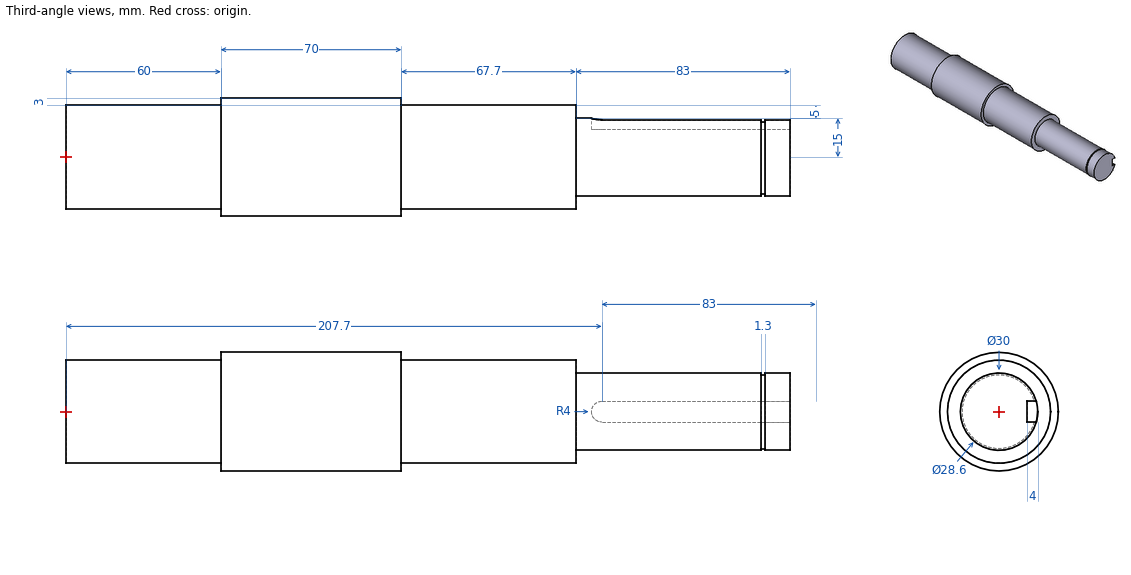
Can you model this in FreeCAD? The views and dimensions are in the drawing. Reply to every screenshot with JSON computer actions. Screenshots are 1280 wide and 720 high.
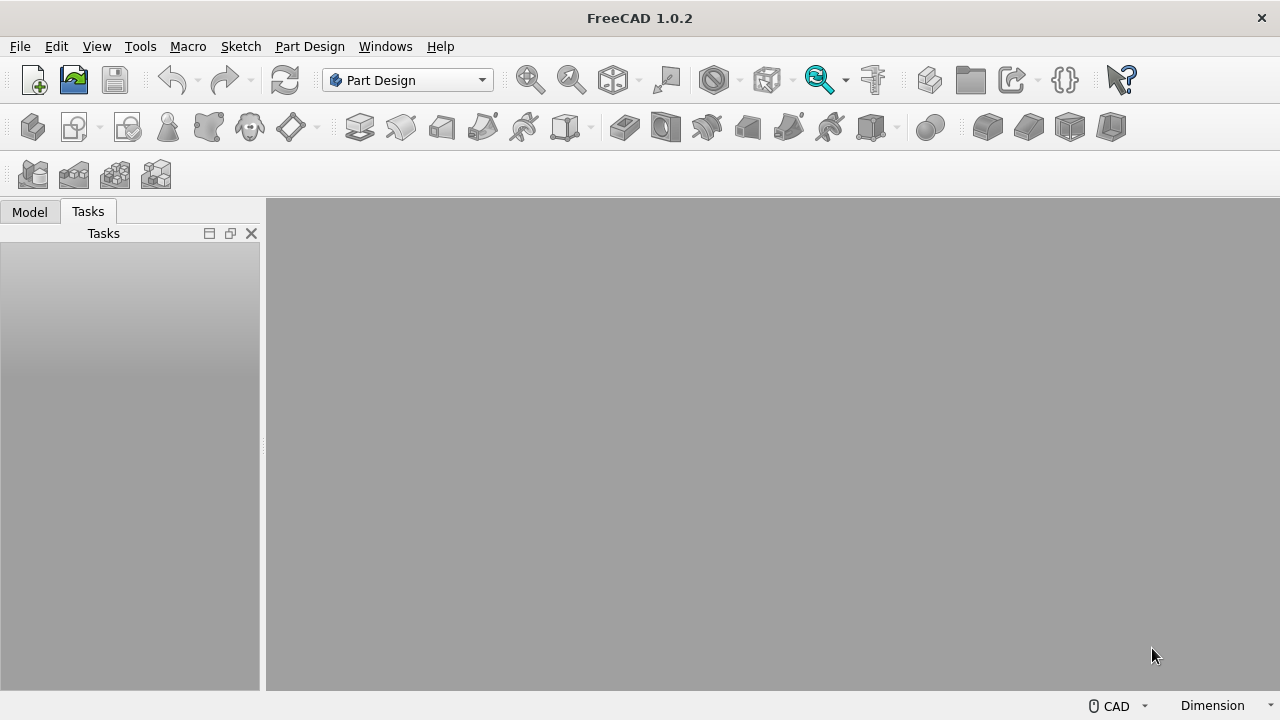
{"action": "key", "text": "ctrl+n"}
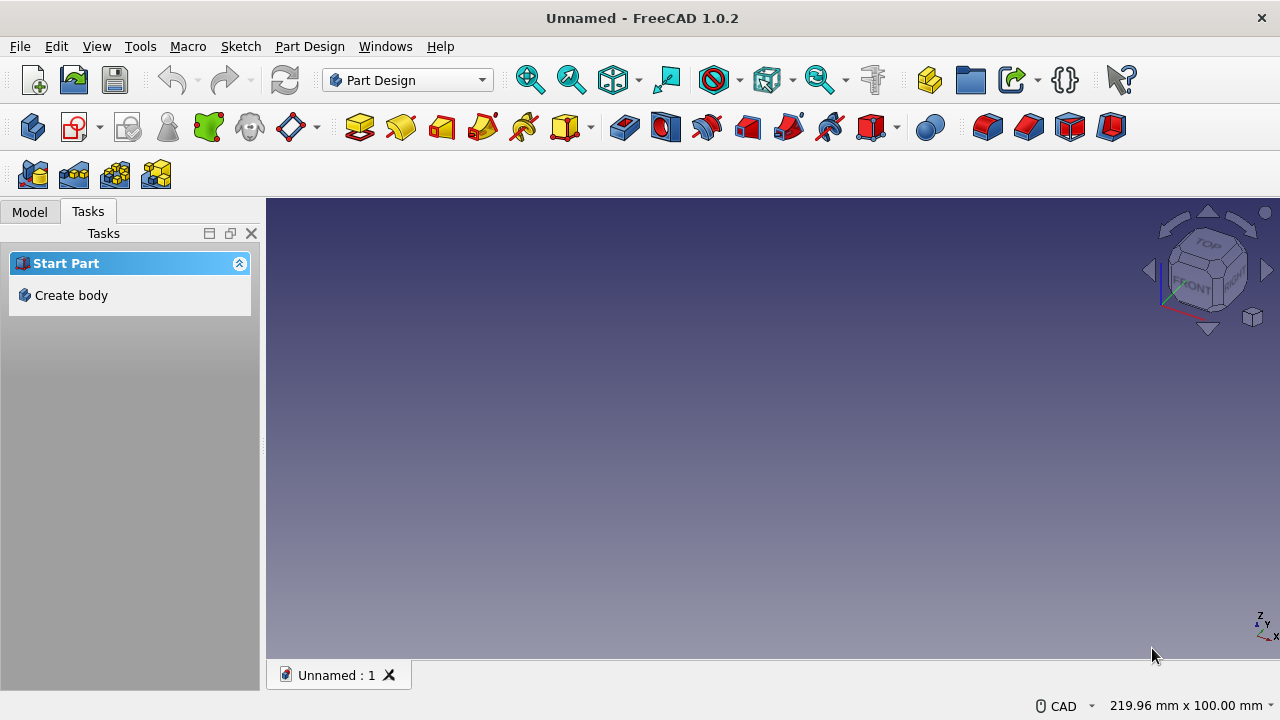
{"action": "left_click", "coordinate": [74, 128]}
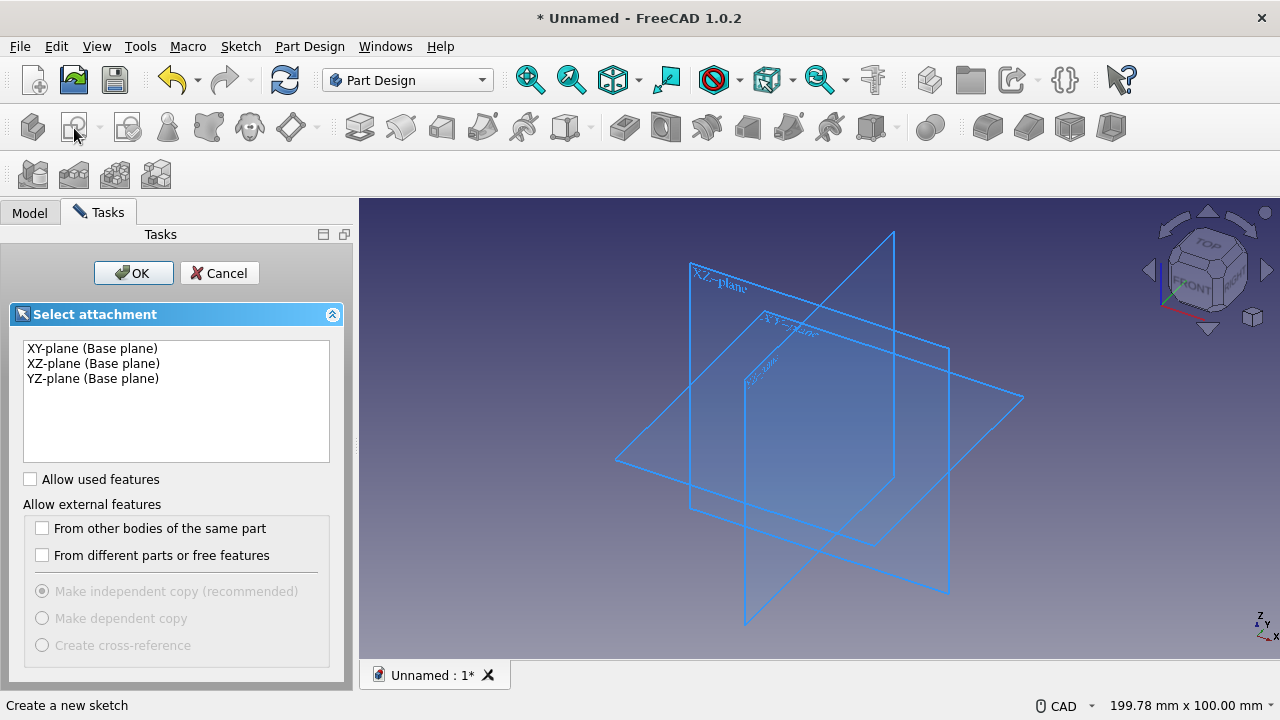
{"action": "left_click", "coordinate": [84, 348]}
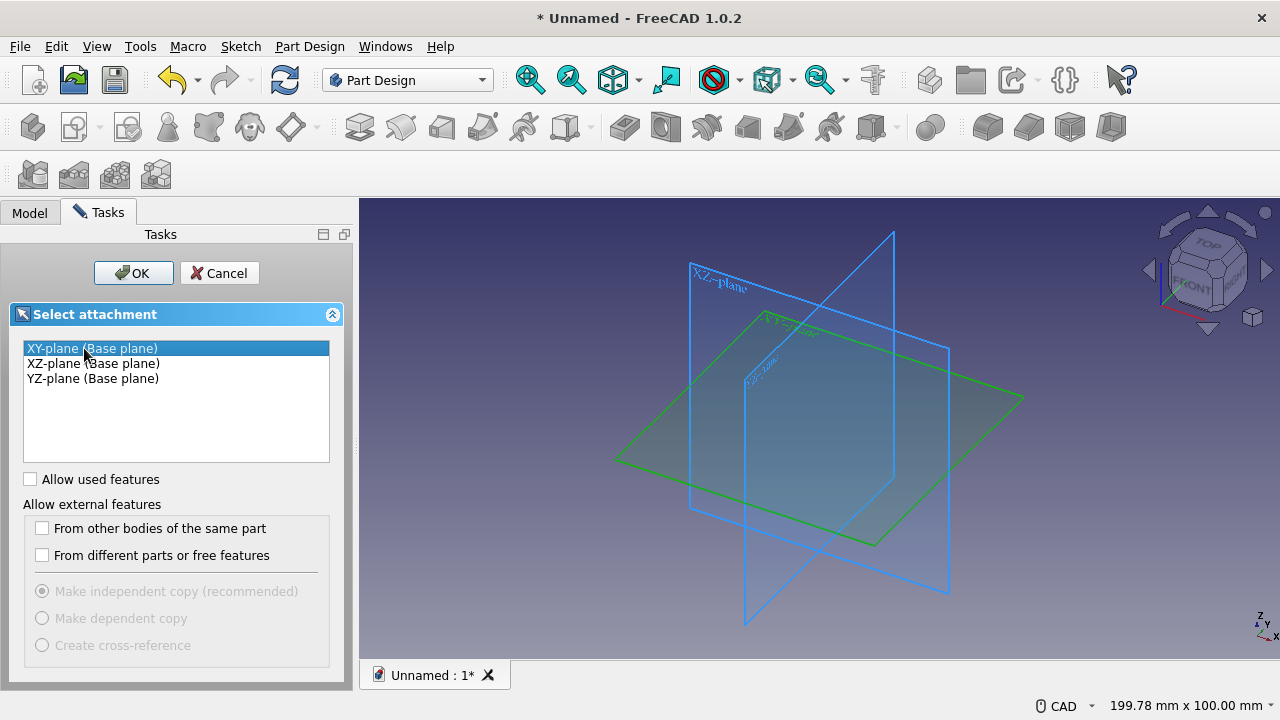
{"action": "left_click", "coordinate": [134, 273]}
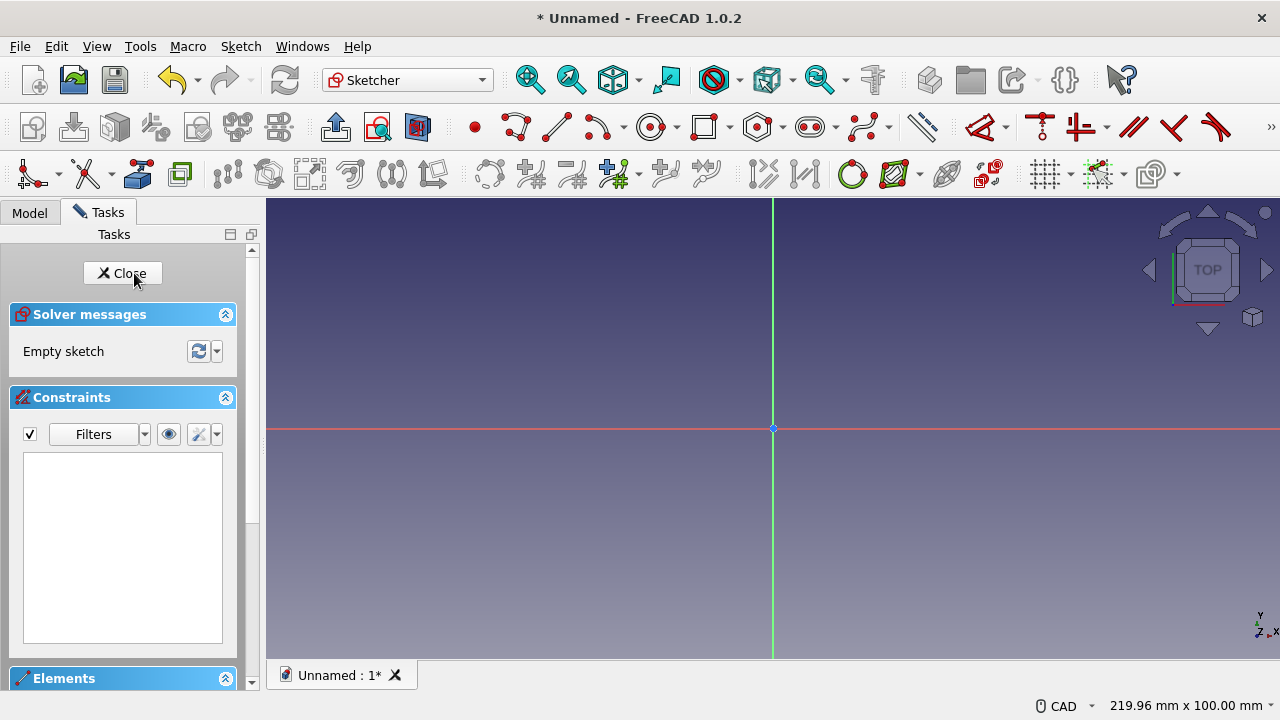
{"action": "scroll", "coordinate": [294, 459], "scroll_direction": "down", "scroll_amount": 5}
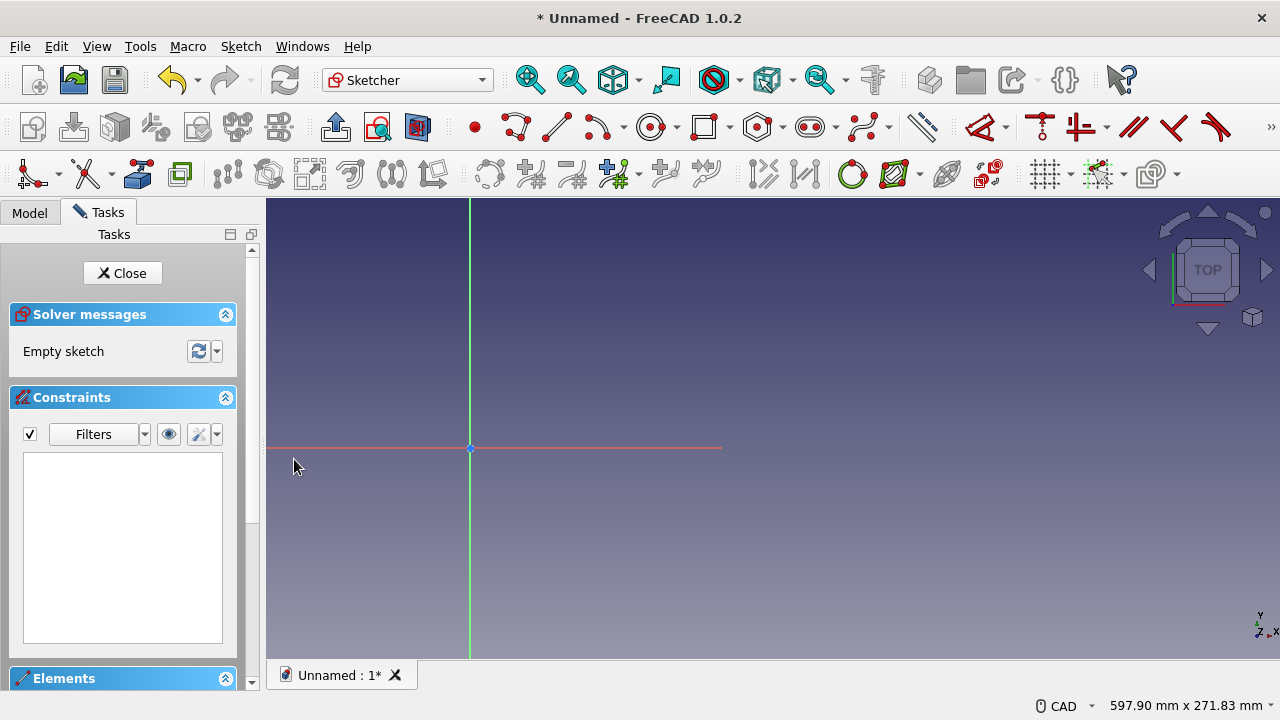
{"action": "key", "text": "g m"}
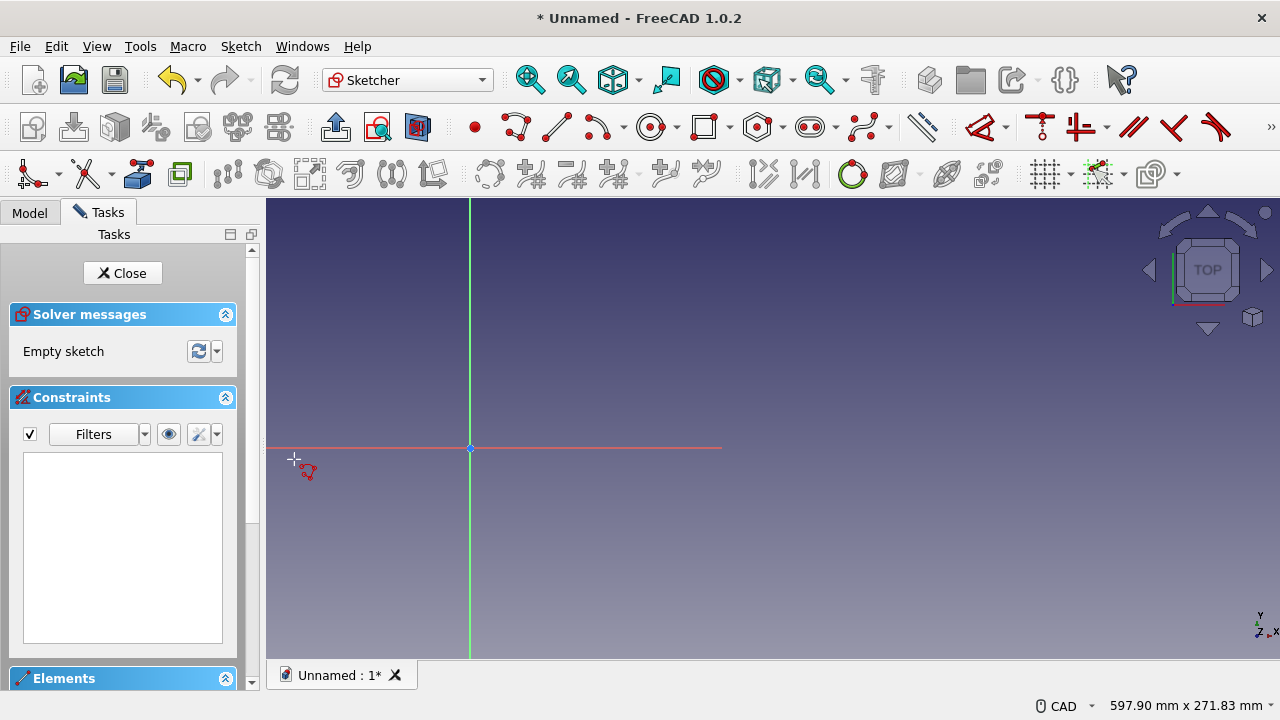
{"action": "left_click", "coordinate": [470, 448]}
{"action": "left_click", "coordinate": [946, 439]}
{"action": "left_click", "coordinate": [946, 423]}
{"action": "left_click", "coordinate": [806, 423]}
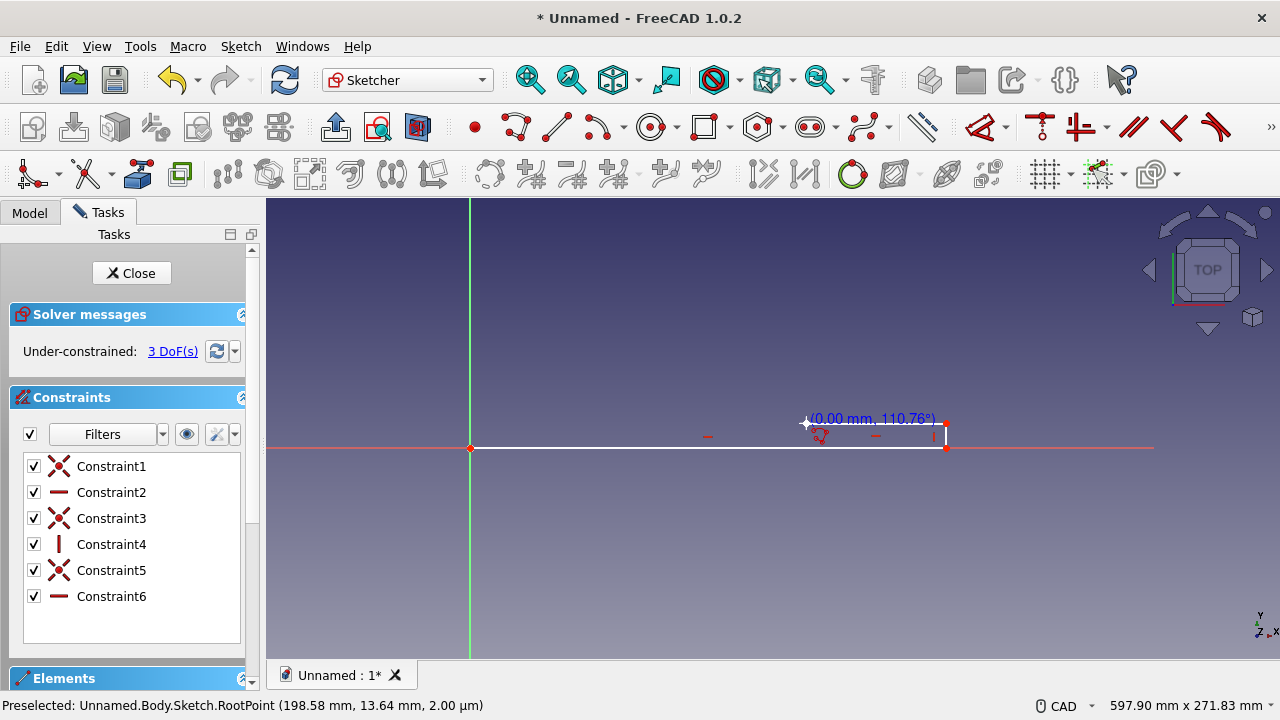
{"action": "scroll", "coordinate": [806, 414], "scroll_direction": "up", "scroll_amount": 4}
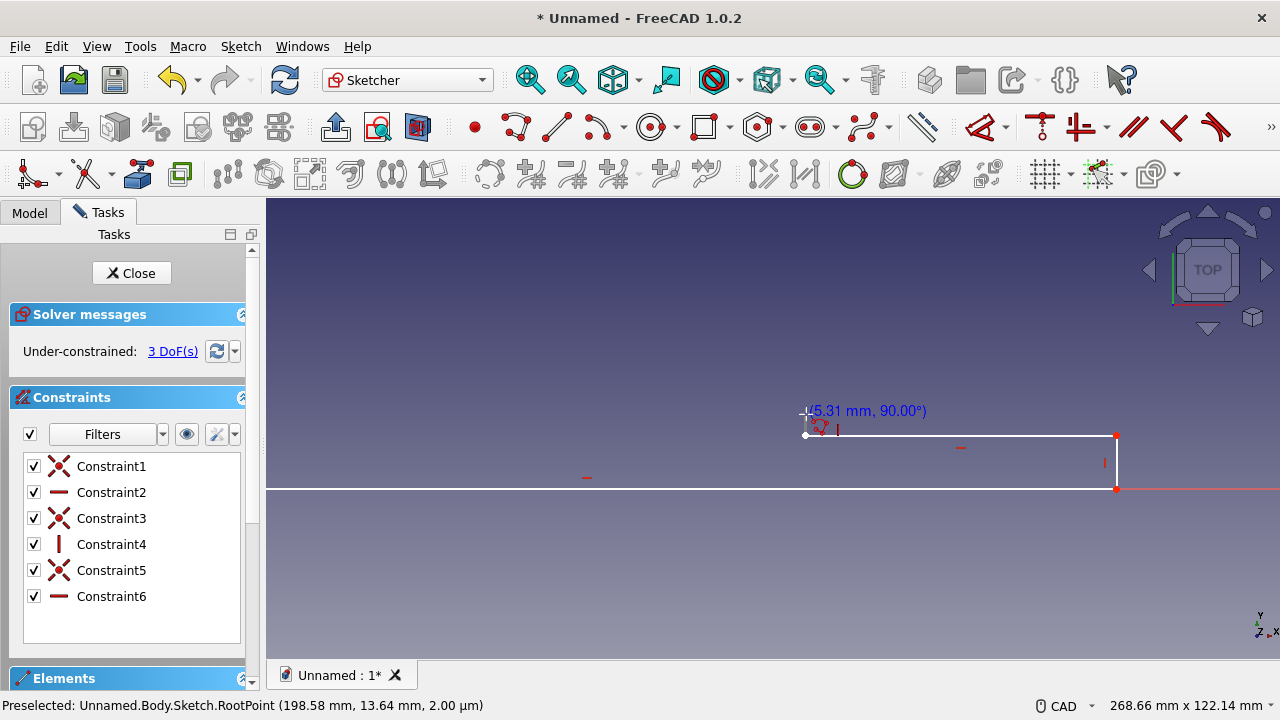
{"action": "left_click", "coordinate": [805, 414]}
{"action": "left_click", "coordinate": [549, 414]}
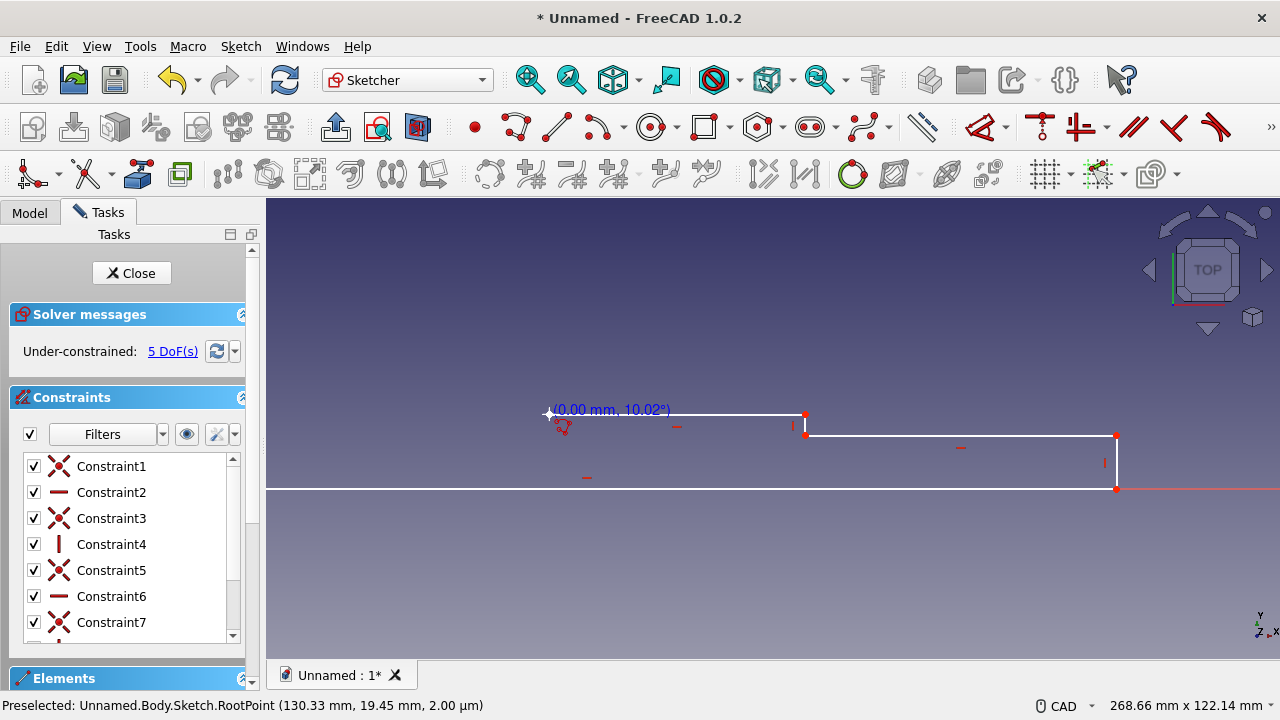
{"action": "scroll", "coordinate": [549, 403], "scroll_direction": "up", "scroll_amount": 2}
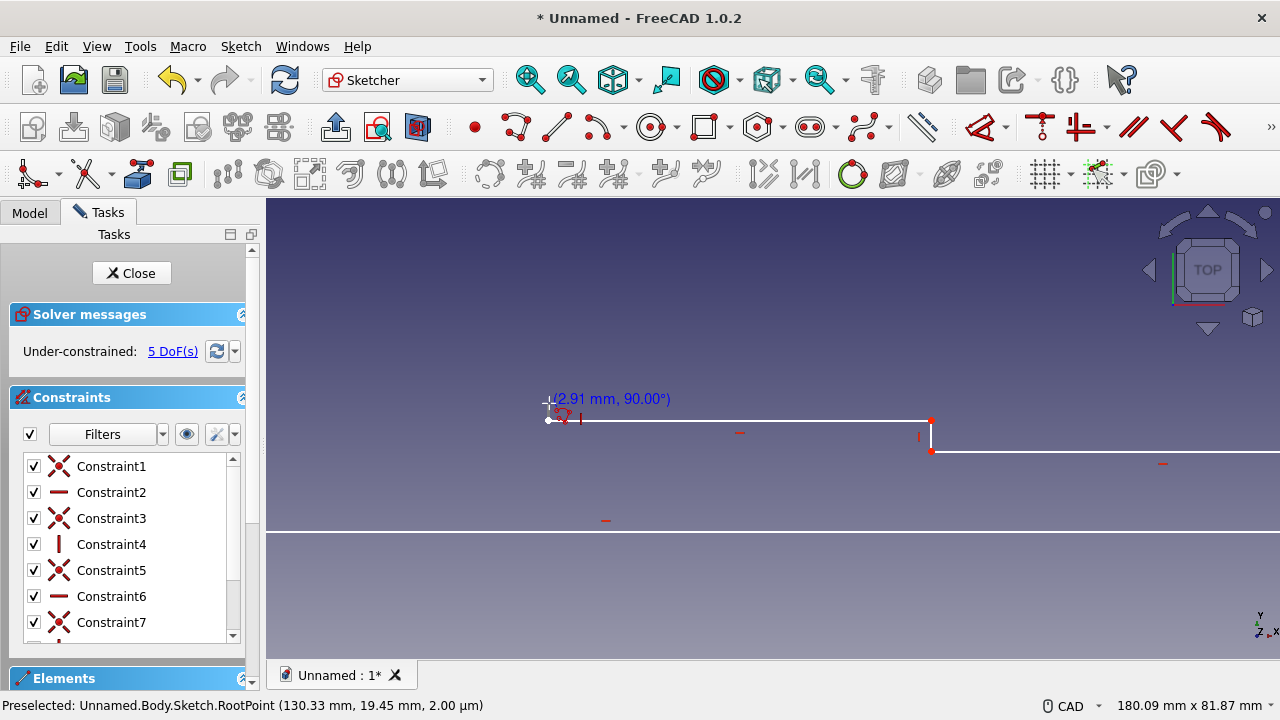
{"action": "left_click", "coordinate": [549, 402]}